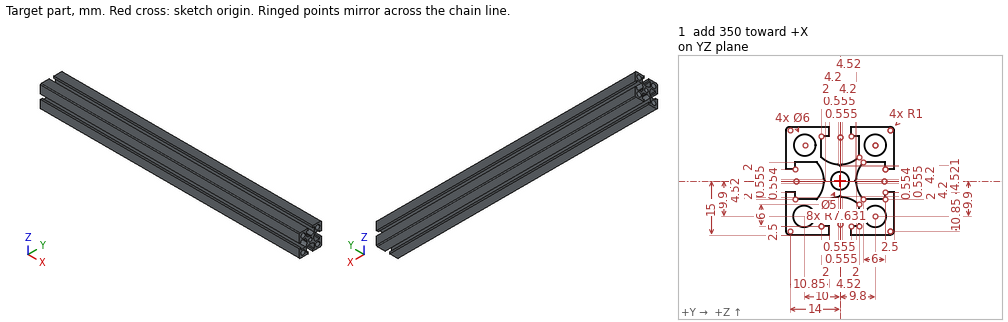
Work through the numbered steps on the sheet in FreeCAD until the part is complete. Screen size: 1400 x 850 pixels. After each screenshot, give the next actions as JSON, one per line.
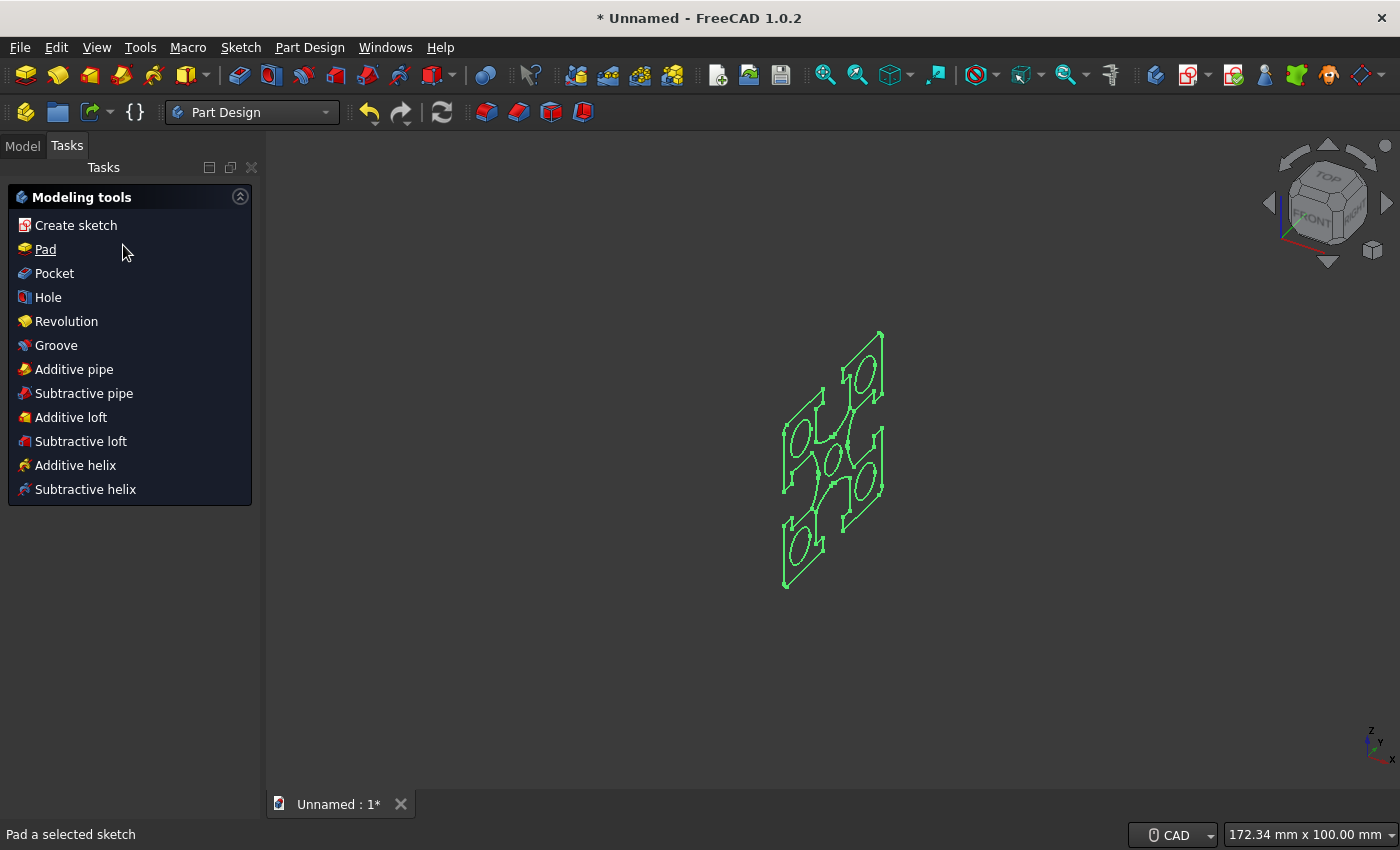
{"action": "left_click", "coordinate": [26, 76]}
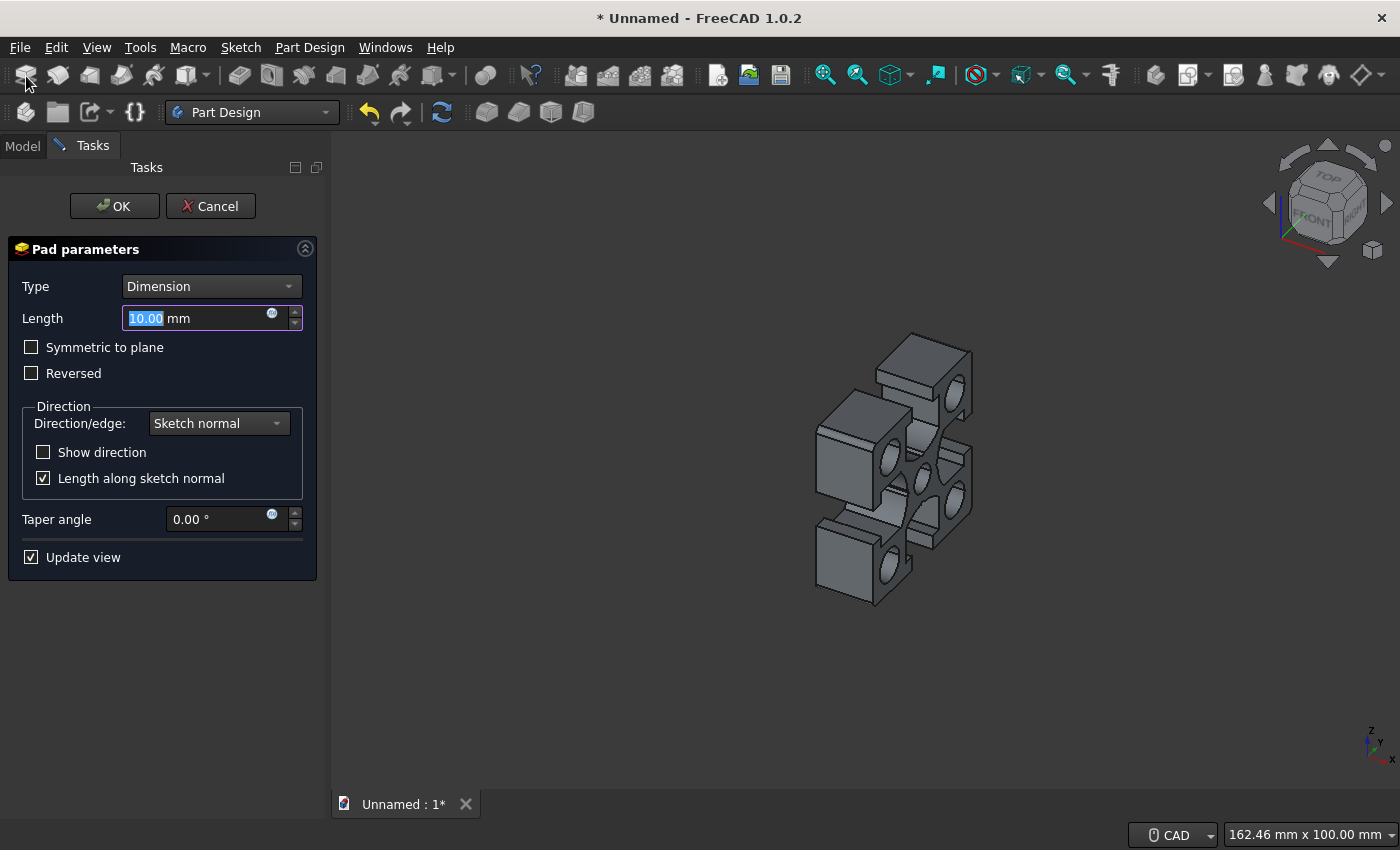
{"action": "type", "text": "350"}
{"action": "key", "text": "Tab"}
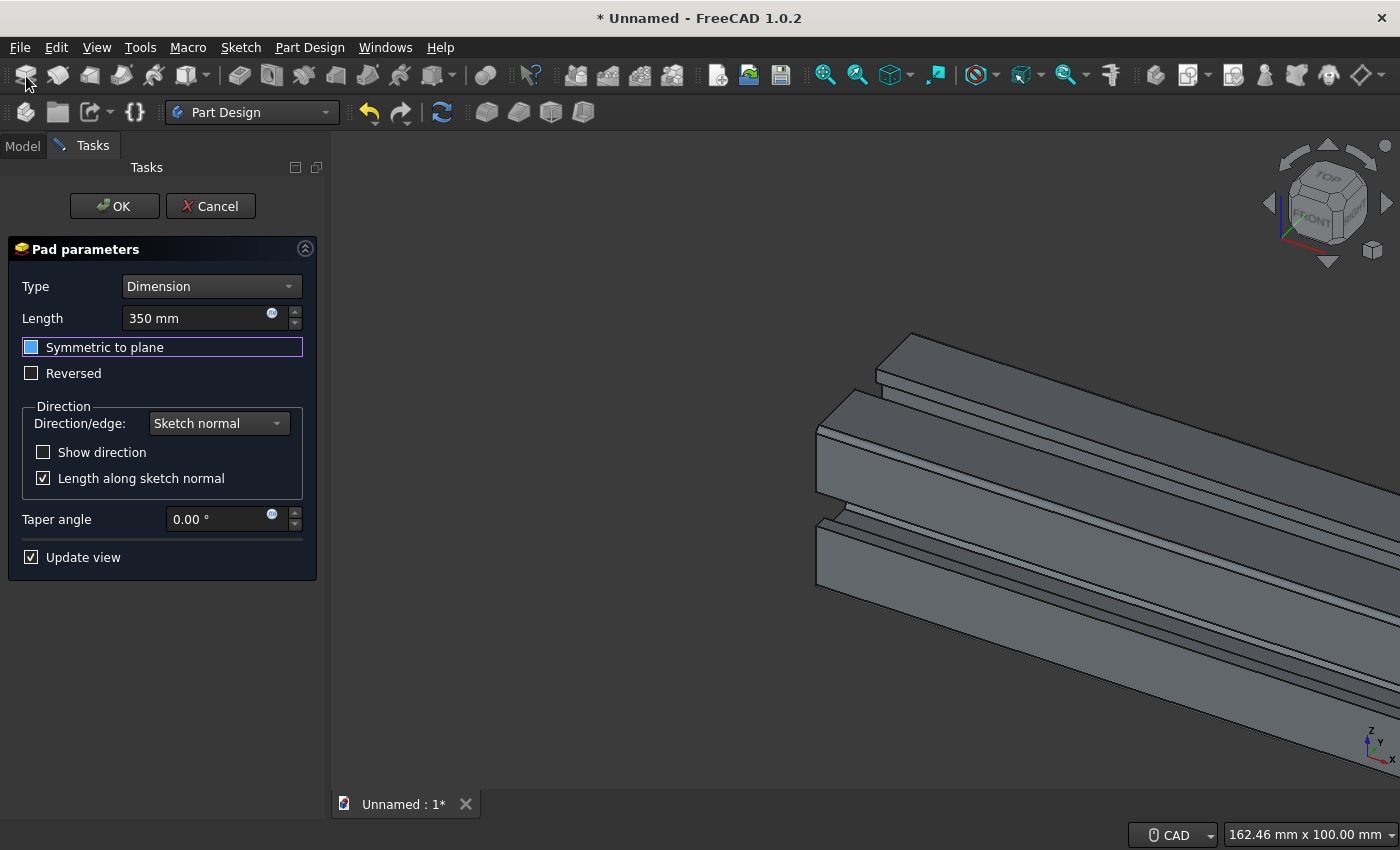
{"action": "left_click", "coordinate": [115, 206]}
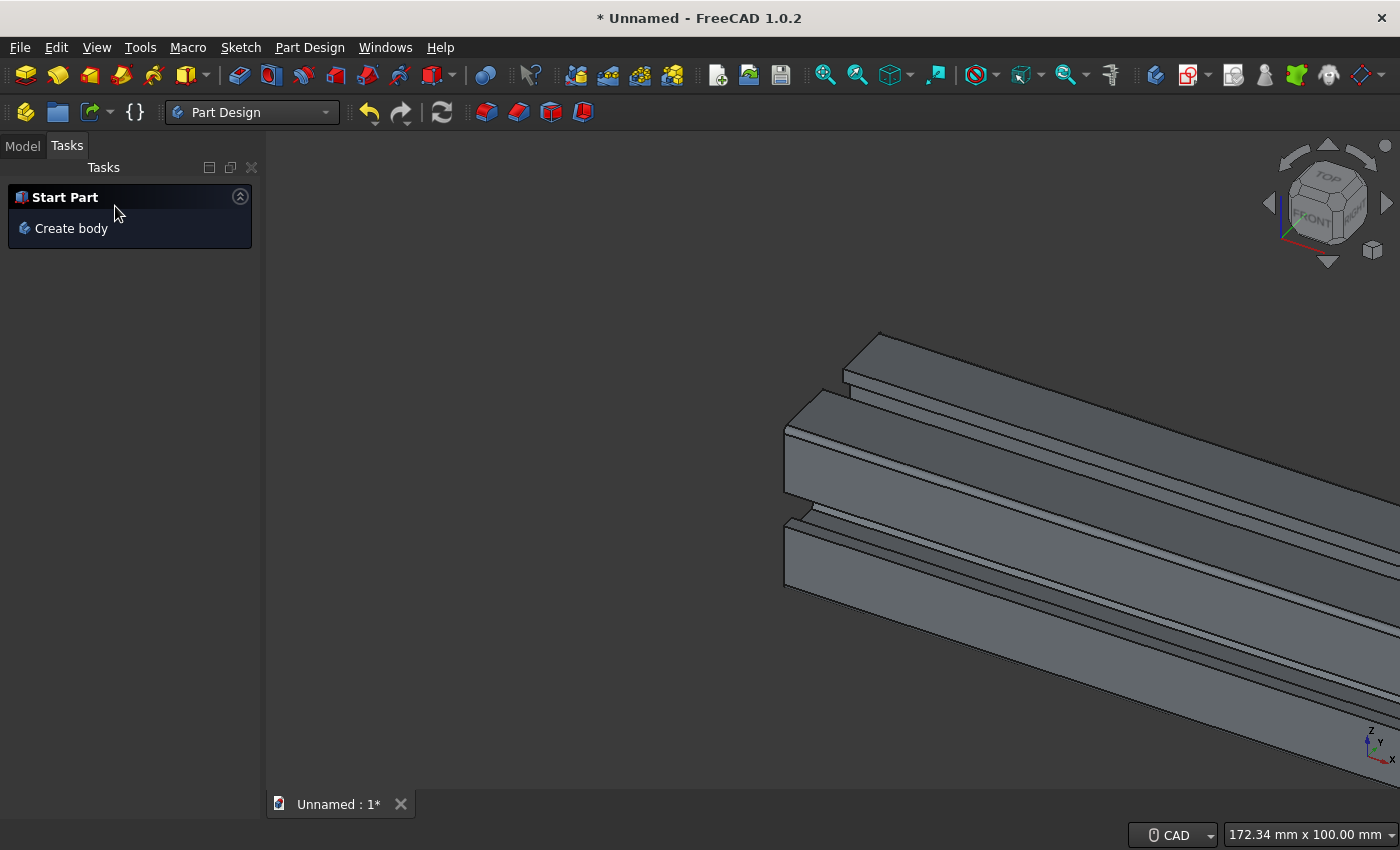
{"action": "key", "text": "0"}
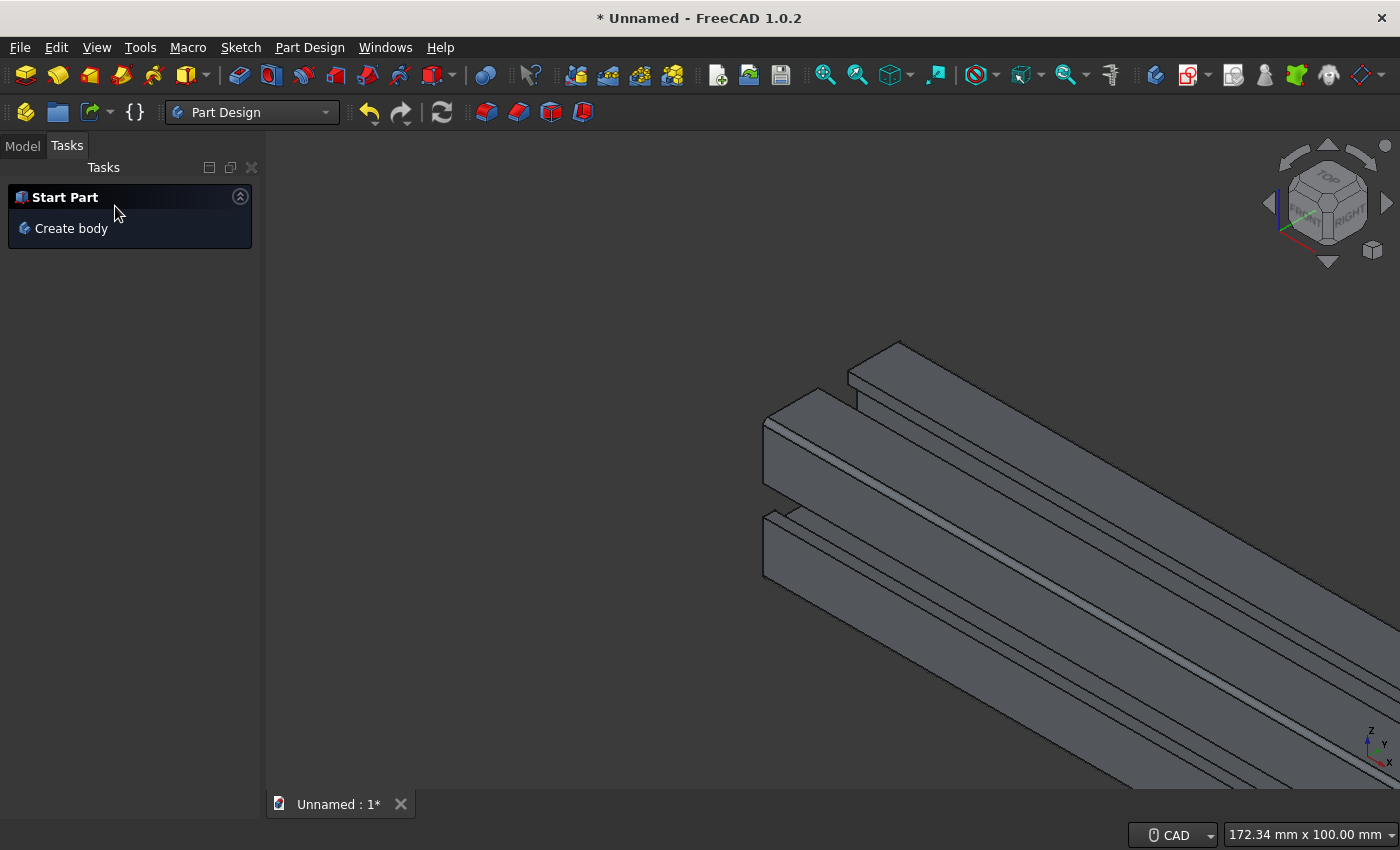
{"action": "left_click", "coordinate": [826, 76]}